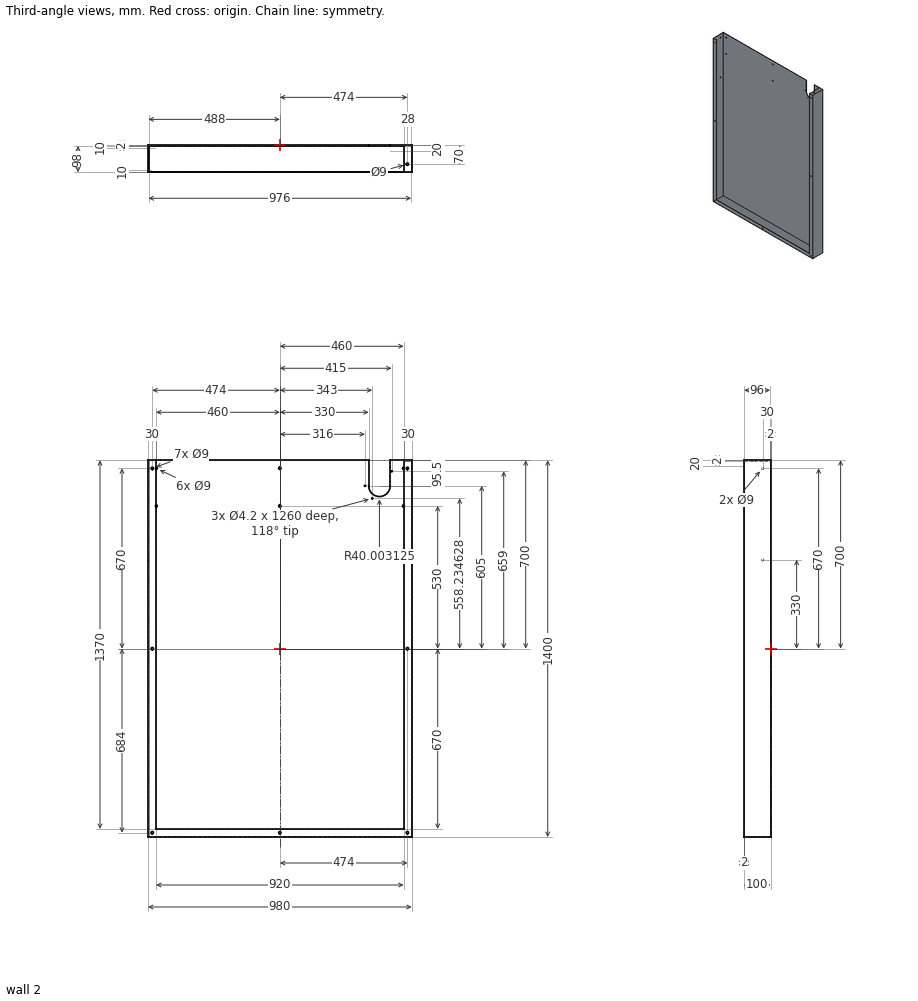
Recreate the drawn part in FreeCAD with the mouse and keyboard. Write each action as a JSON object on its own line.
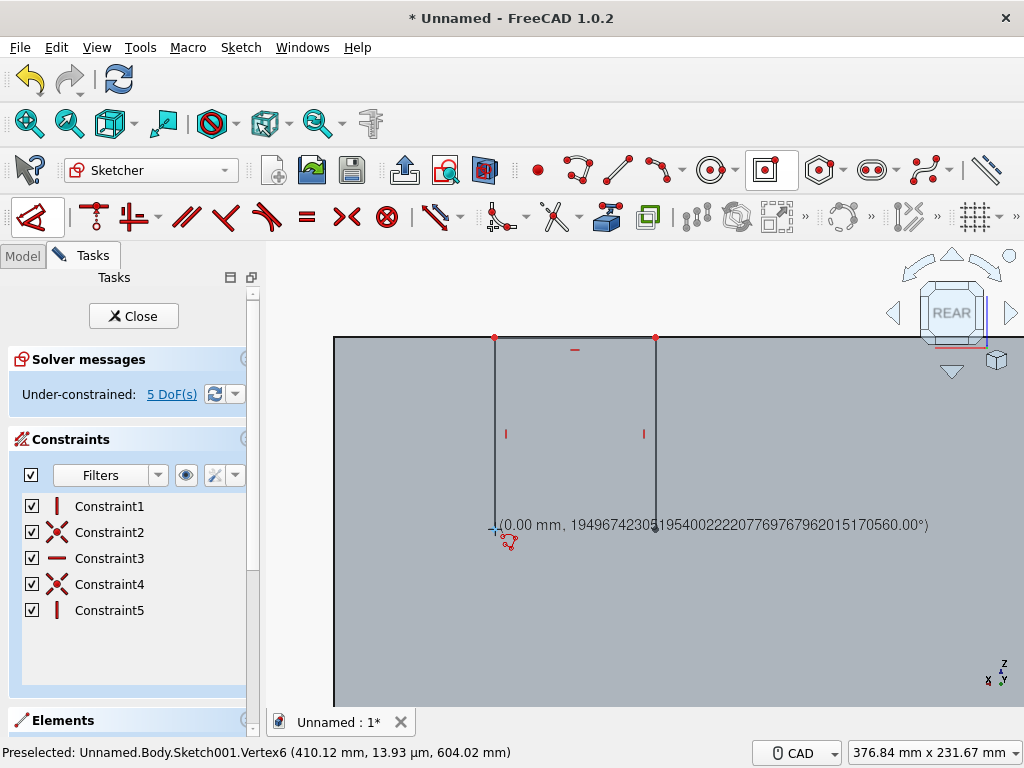
{"action": "left_click", "coordinate": [658, 170]}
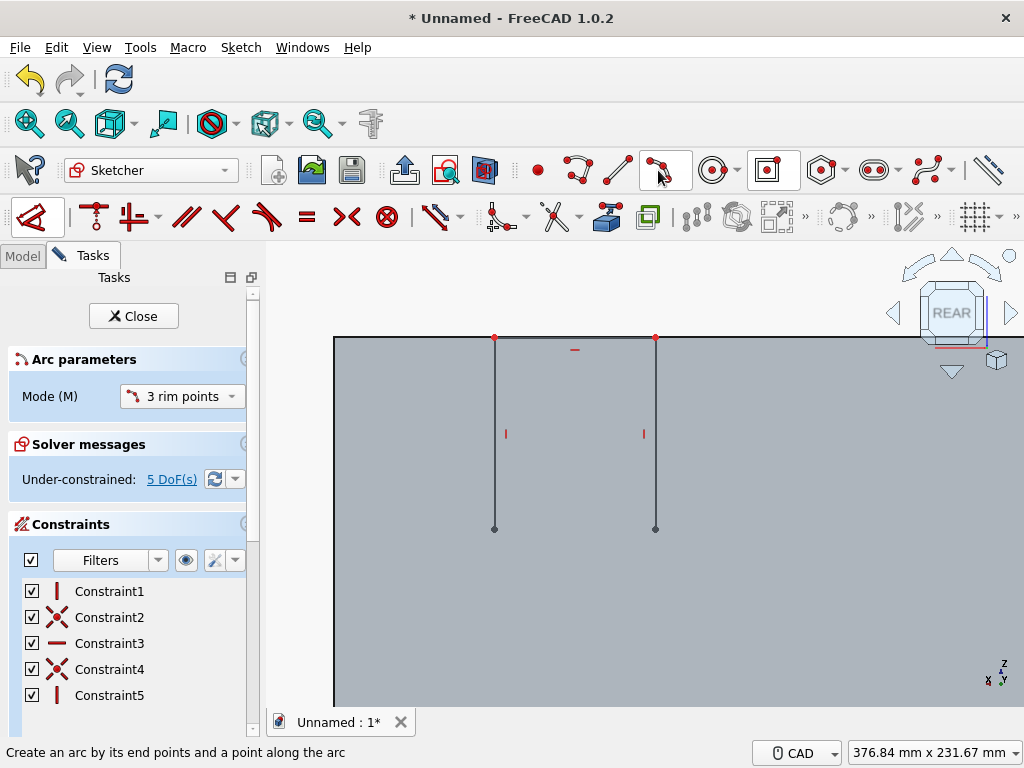
{"action": "left_click", "coordinate": [495, 530]}
{"action": "left_click", "coordinate": [656, 530]}
{"action": "left_click", "coordinate": [576, 608]}
{"action": "key", "text": "Escape"}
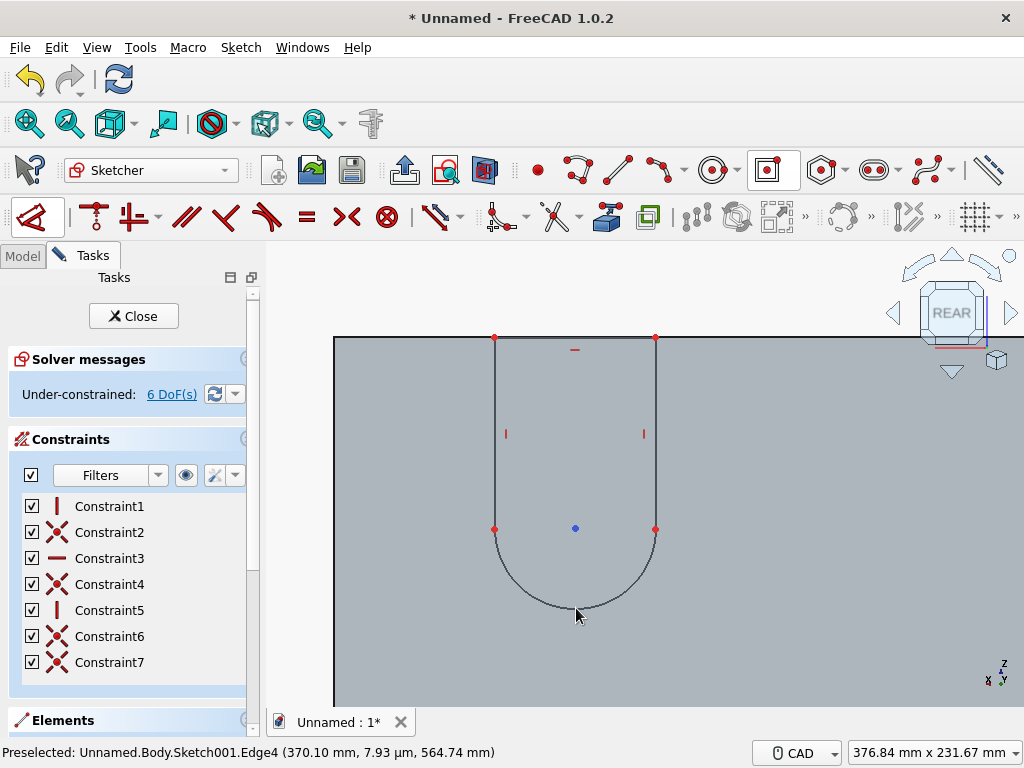
{"action": "left_click", "coordinate": [529, 594]}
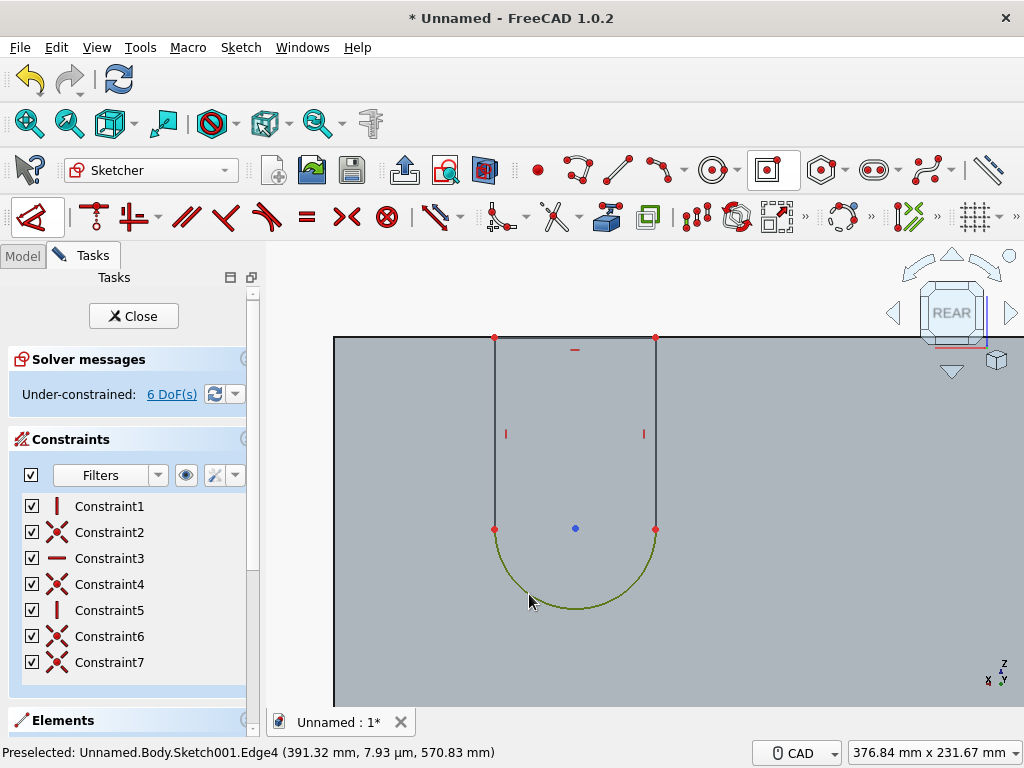
{"action": "key", "text": "k r"}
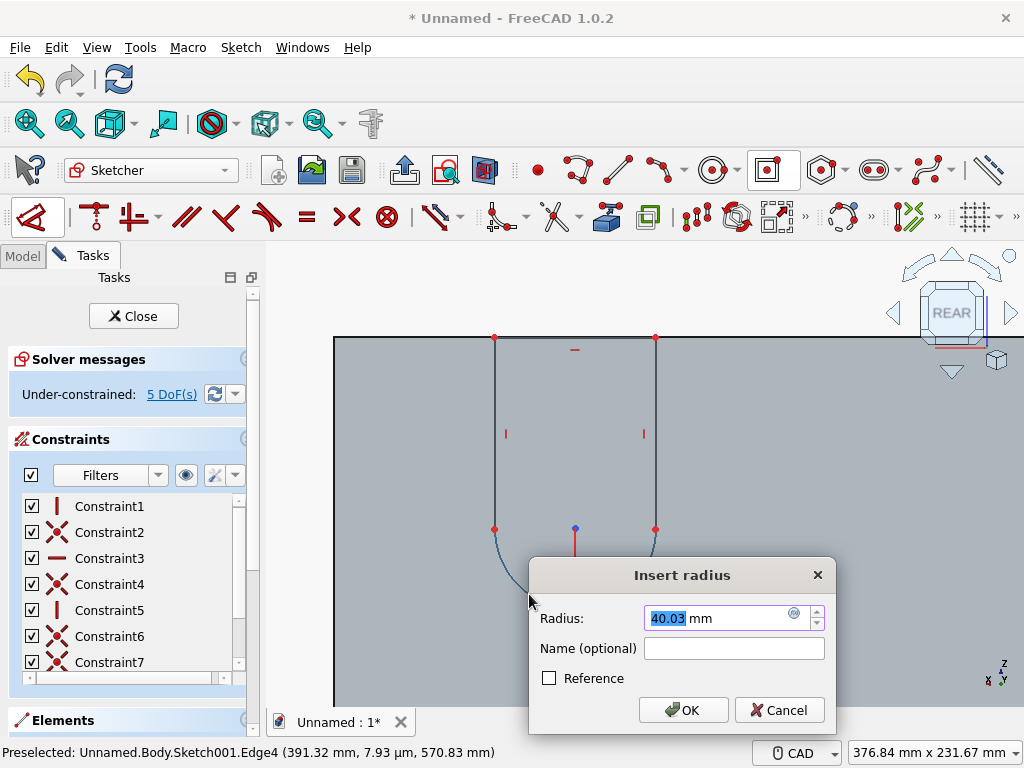
{"action": "type", "text": "40.003125"}
{"action": "key", "text": "Return"}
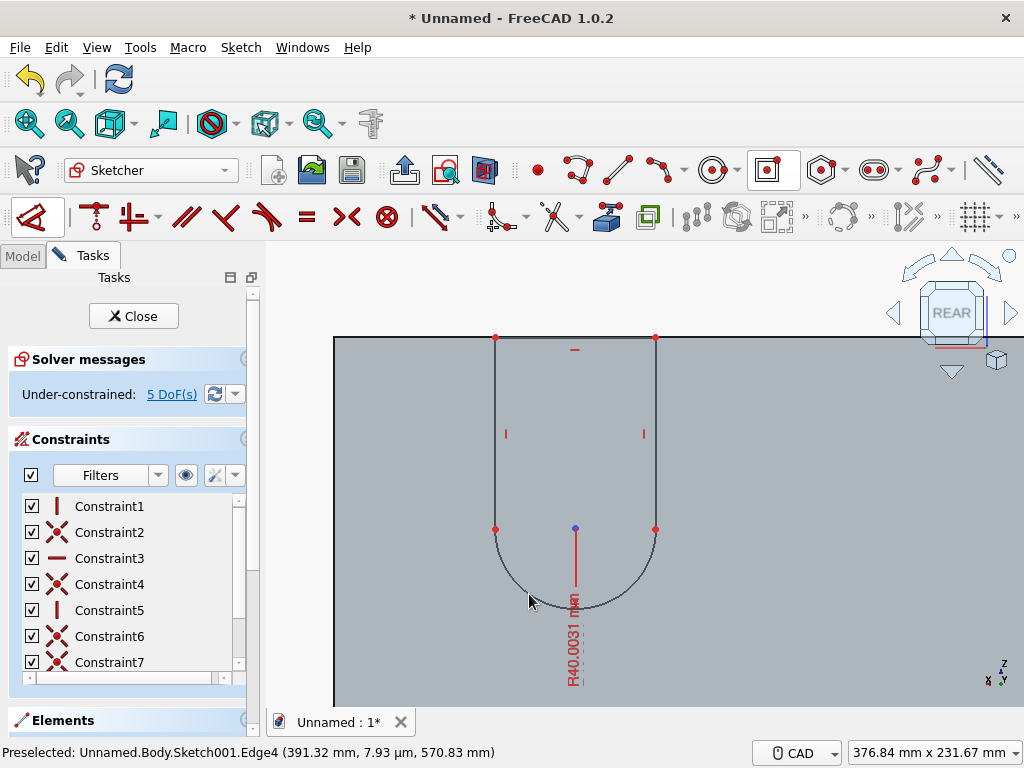
{"action": "left_click", "coordinate": [656, 472]}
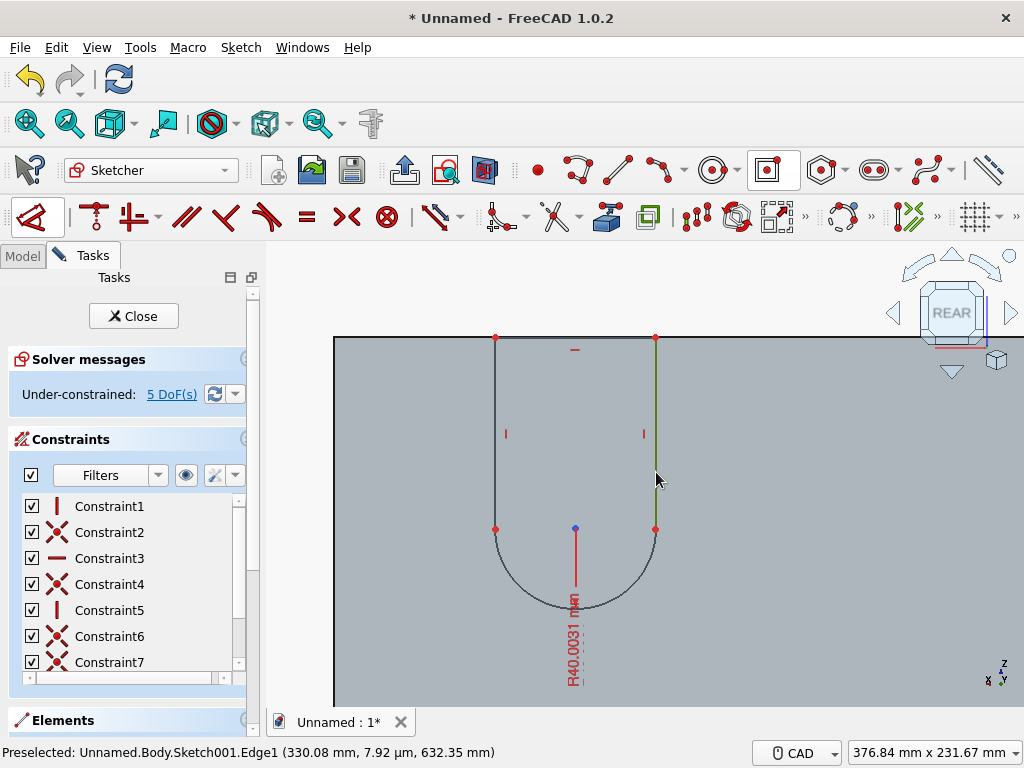
{"action": "key", "text": "i"}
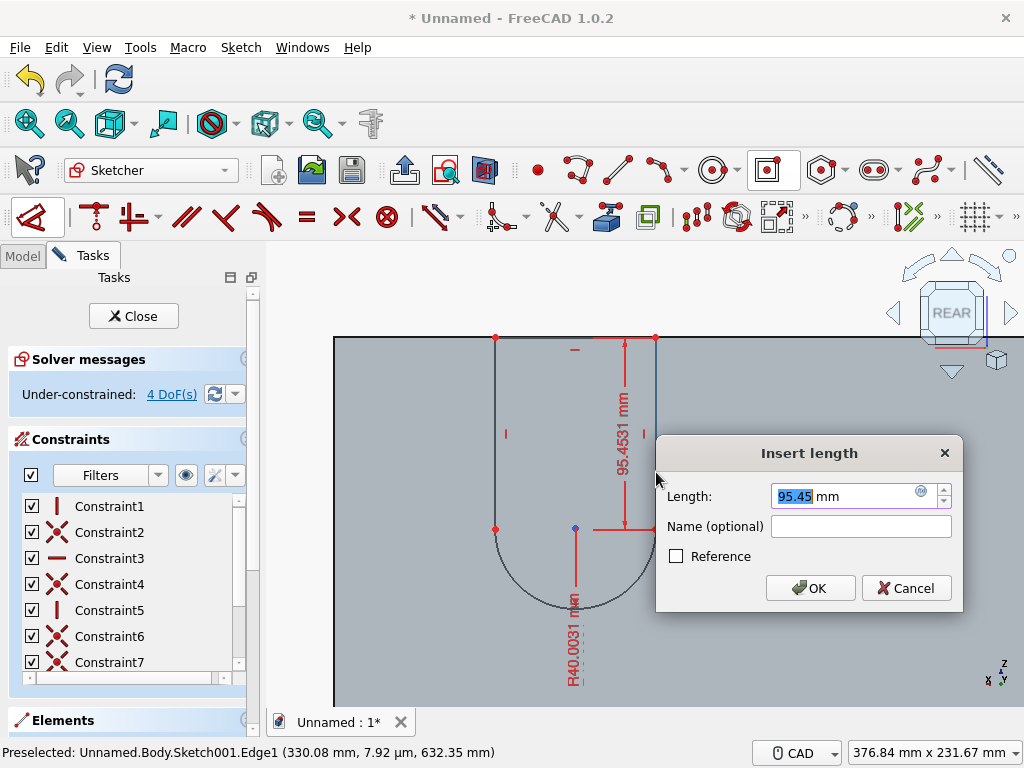
{"action": "type", "text": "95.5"}
{"action": "key", "text": "Return"}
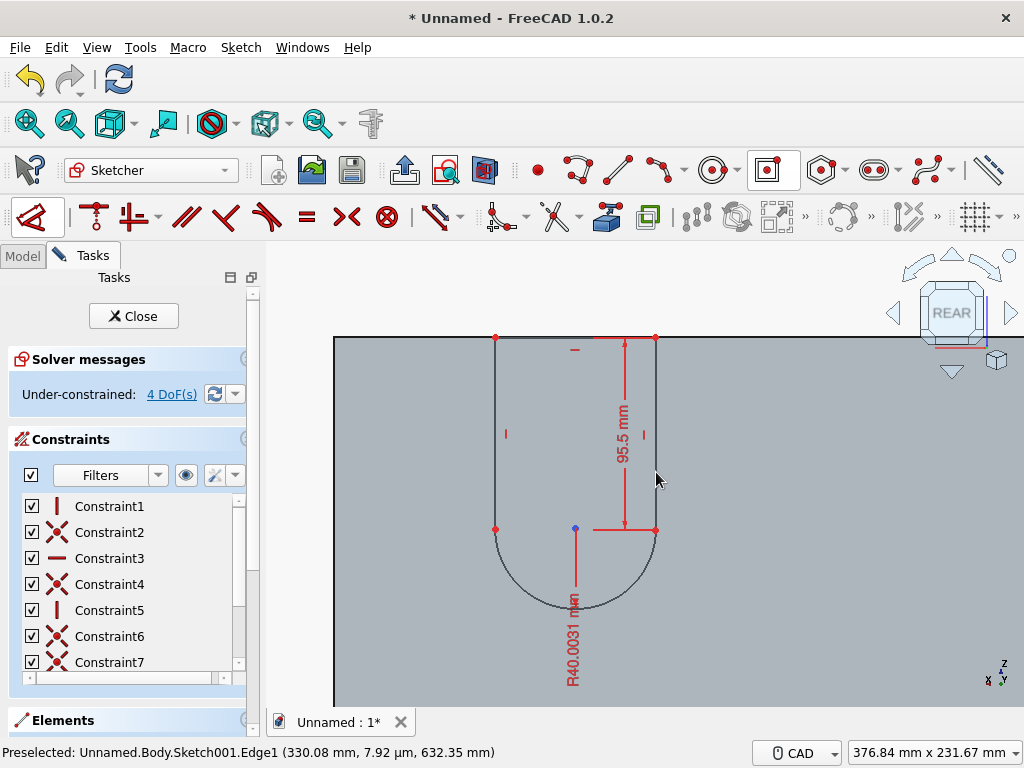
{"action": "left_click", "coordinate": [495, 396]}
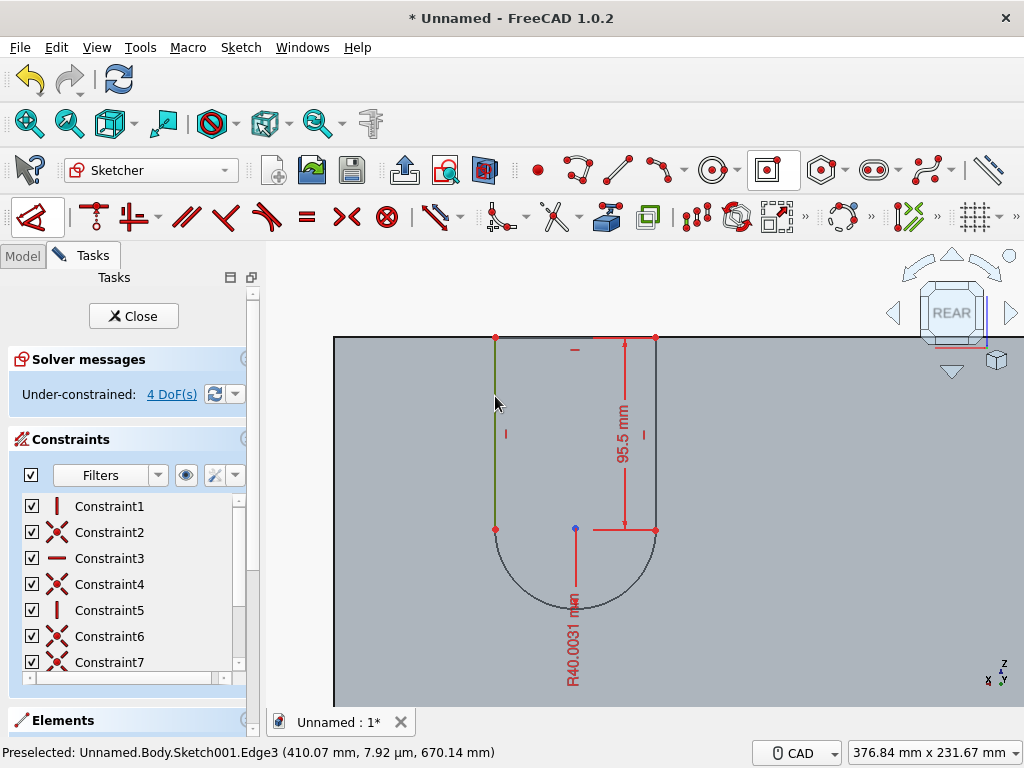
{"action": "left_click", "coordinate": [58, 218]}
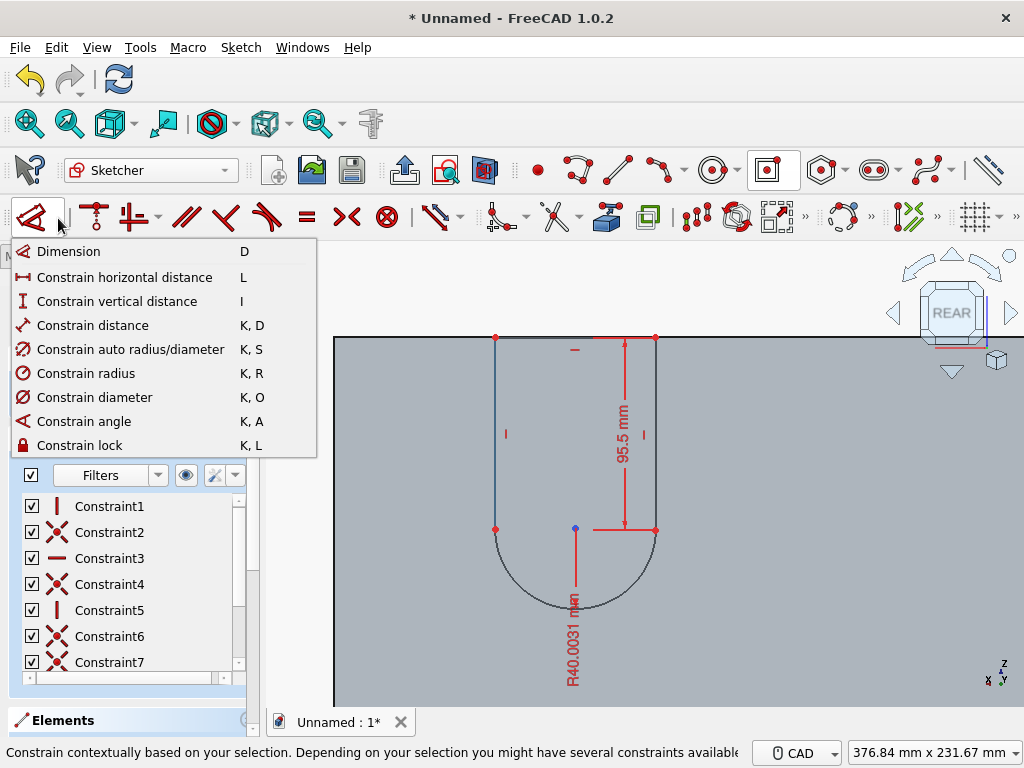
{"action": "left_click", "coordinate": [164, 301]}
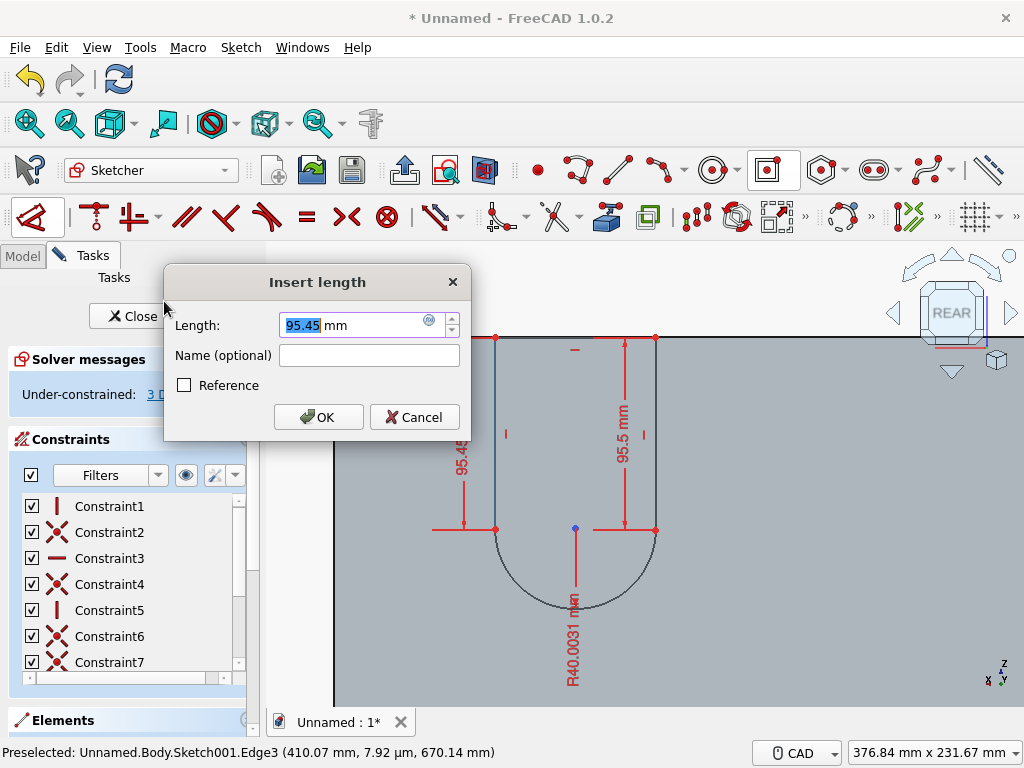
{"action": "type", "text": "95.5"}
{"action": "key", "text": "Return"}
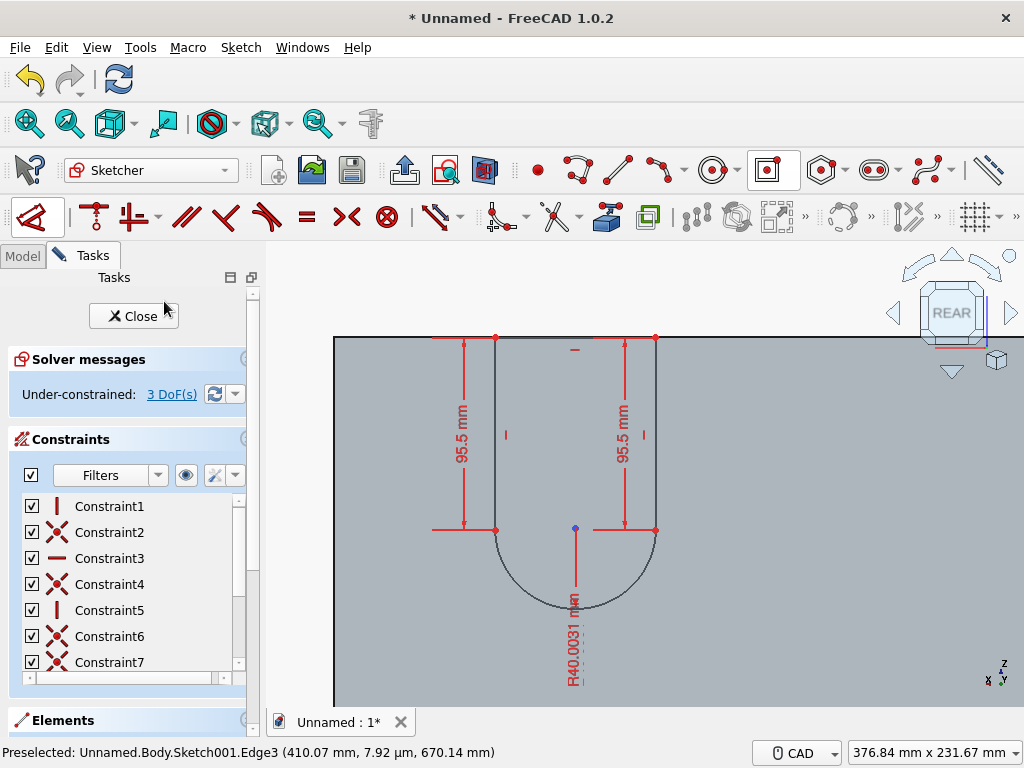
{"action": "left_click", "coordinate": [656, 530]}